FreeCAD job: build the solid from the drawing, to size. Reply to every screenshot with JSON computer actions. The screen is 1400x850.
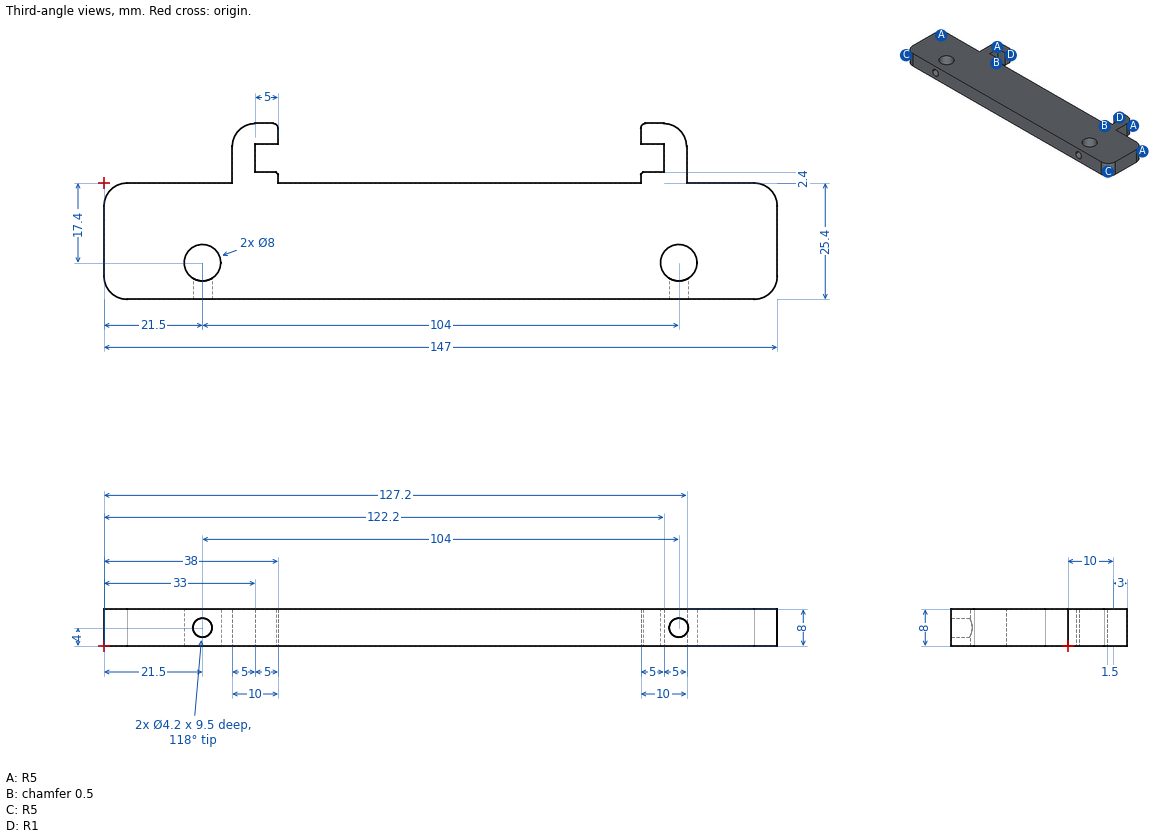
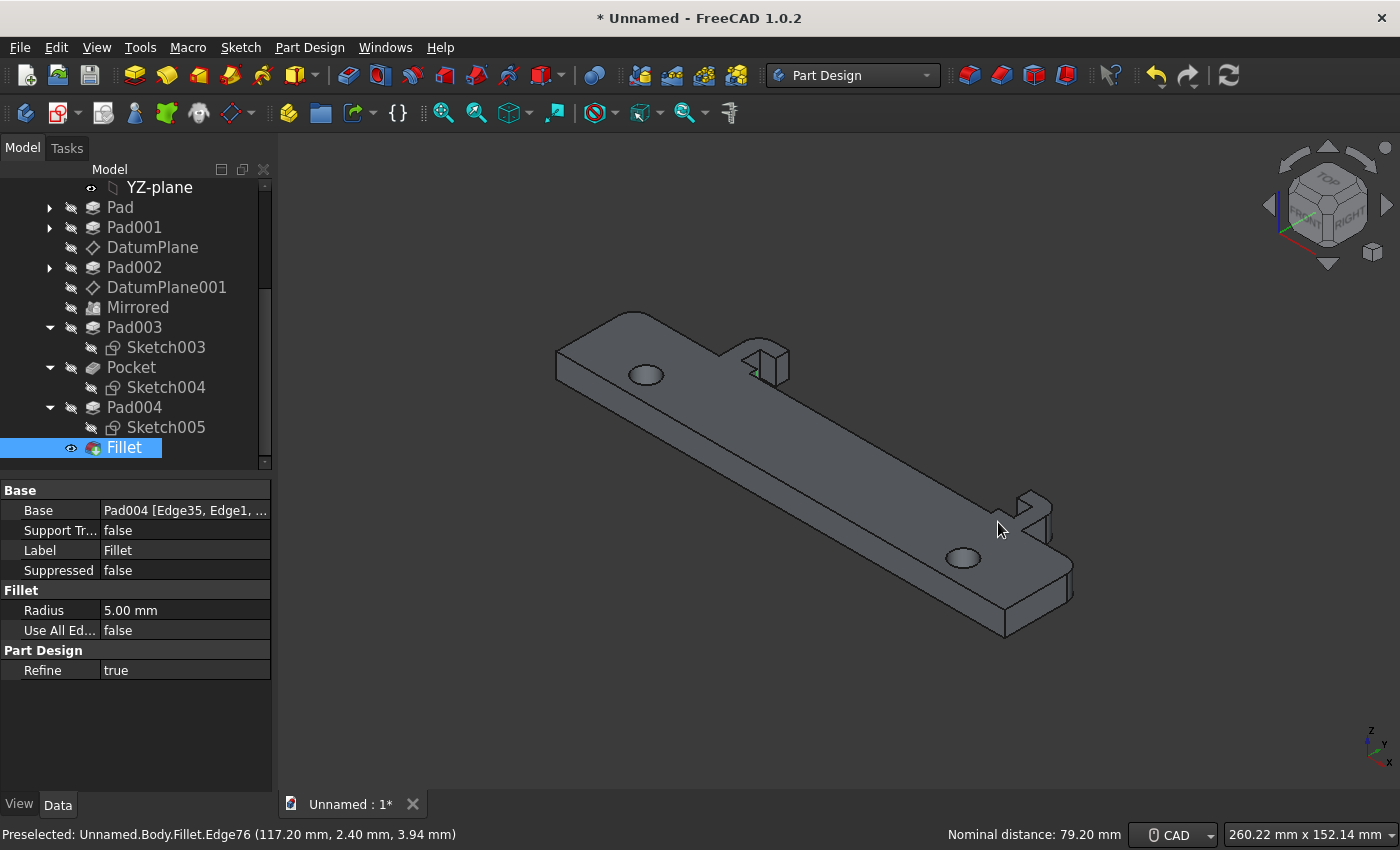
{"action": "left_click", "coordinate": [1002, 76]}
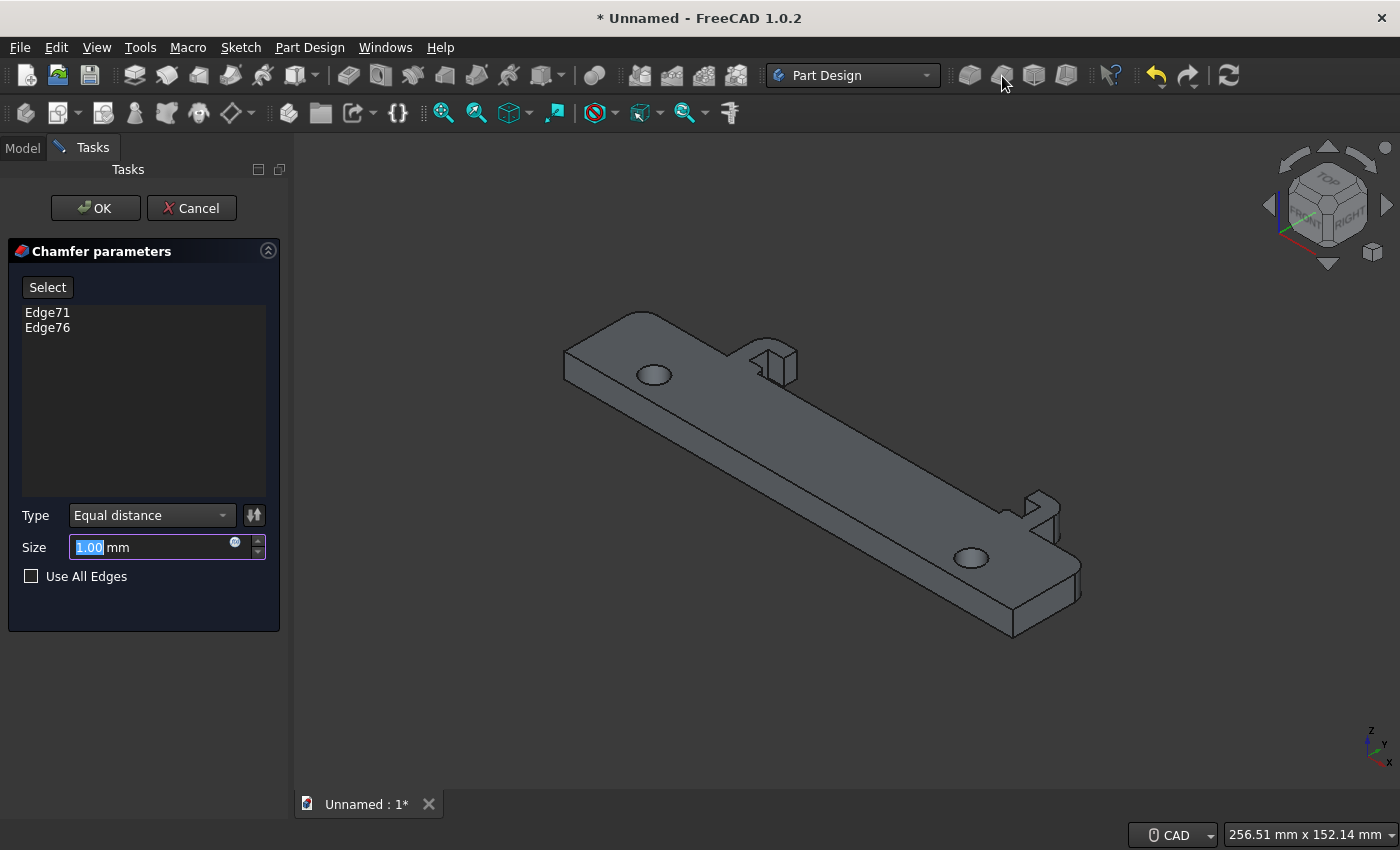
{"action": "type", "text": "0.5"}
{"action": "key", "text": "Tab"}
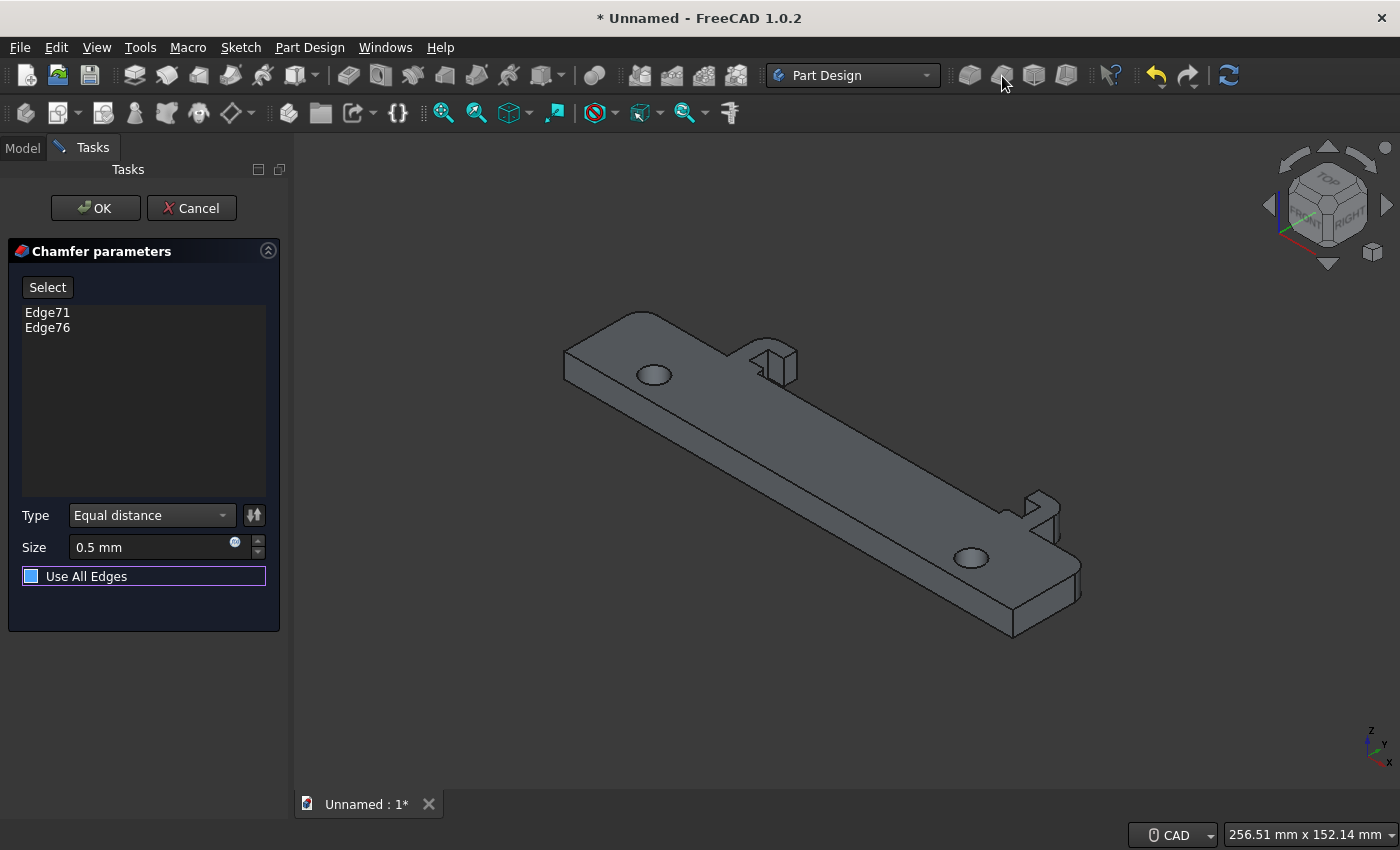
{"action": "left_click", "coordinate": [96, 208]}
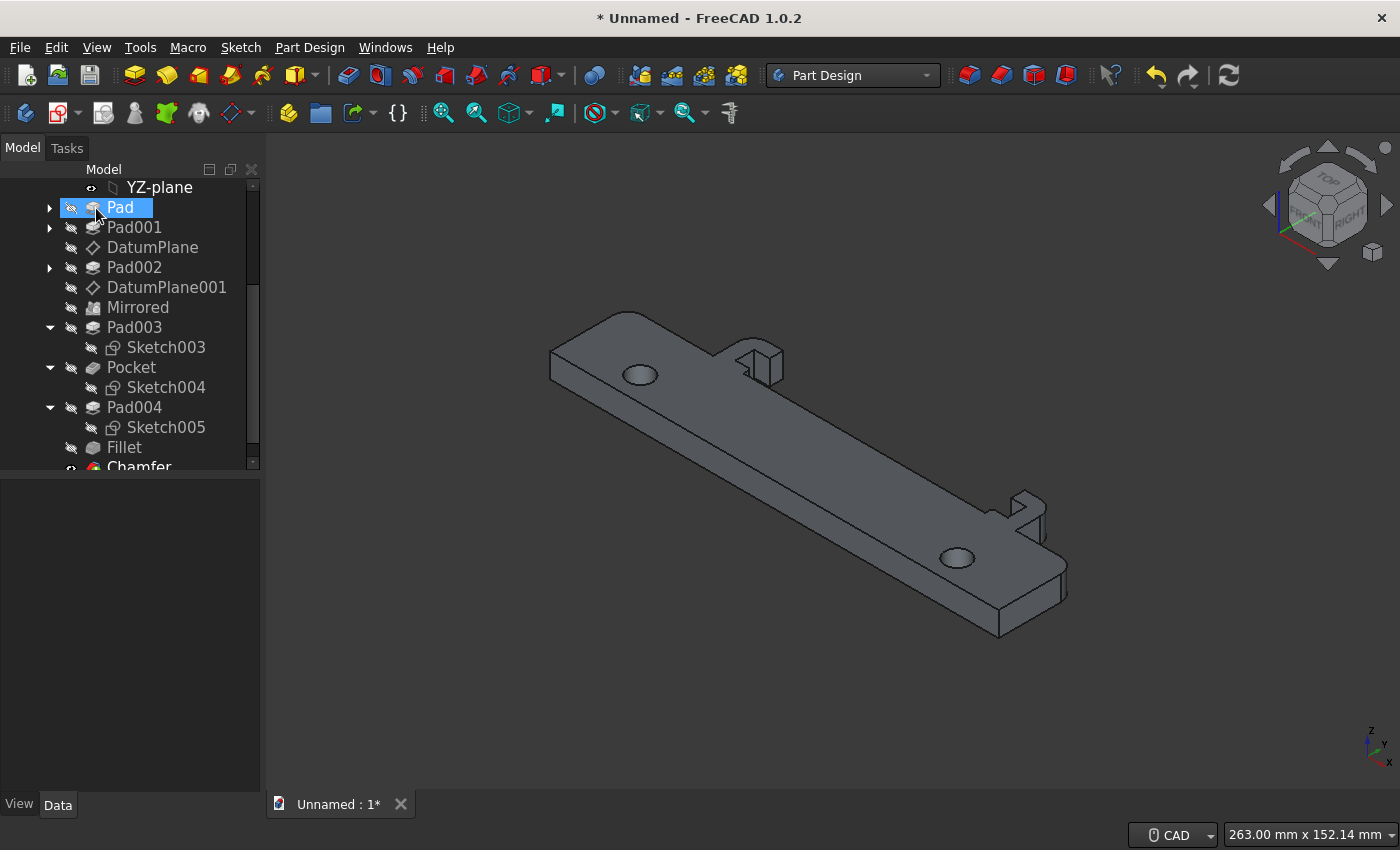
{"action": "left_click", "coordinate": [967, 605]}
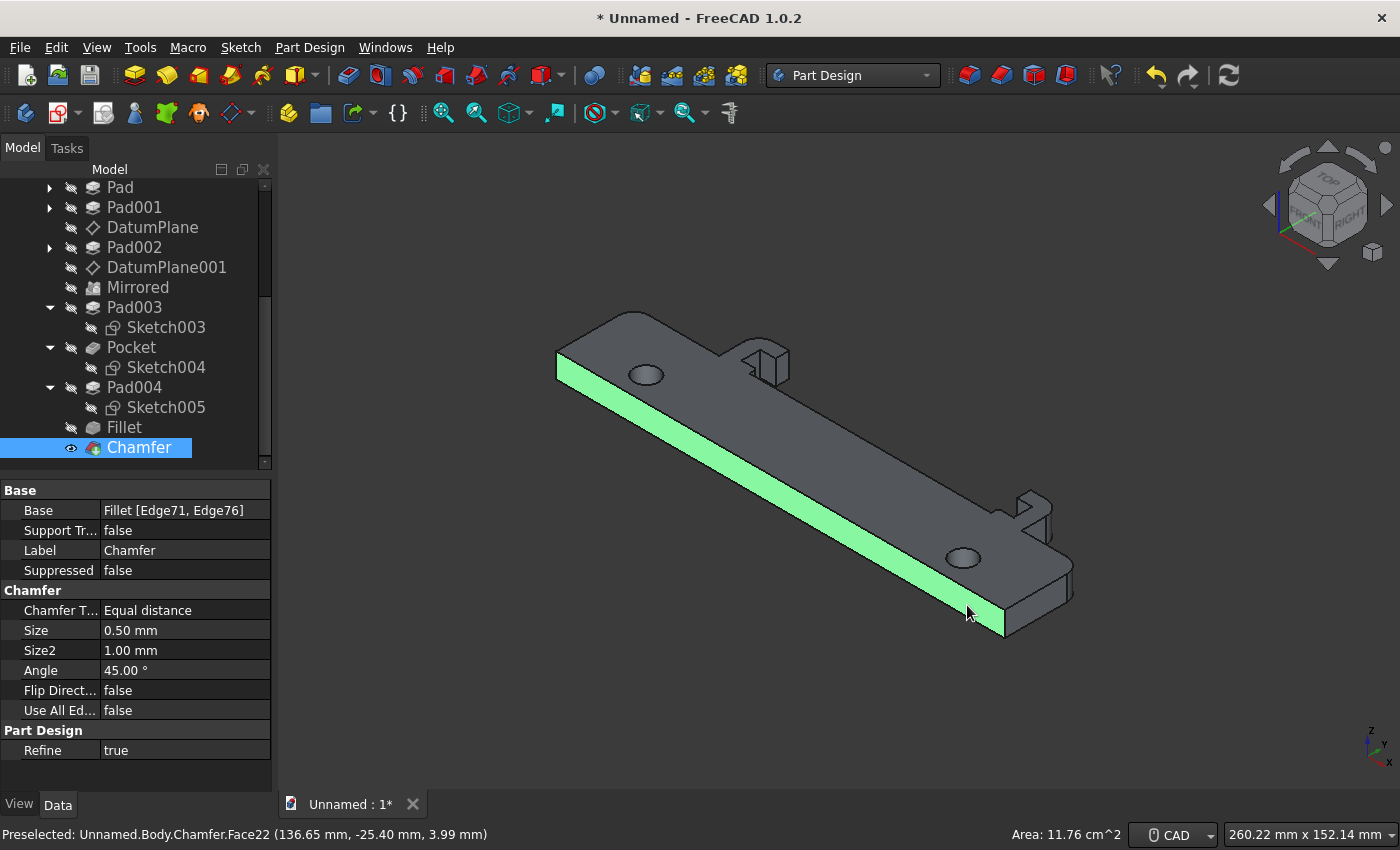
{"action": "left_click", "coordinate": [58, 114]}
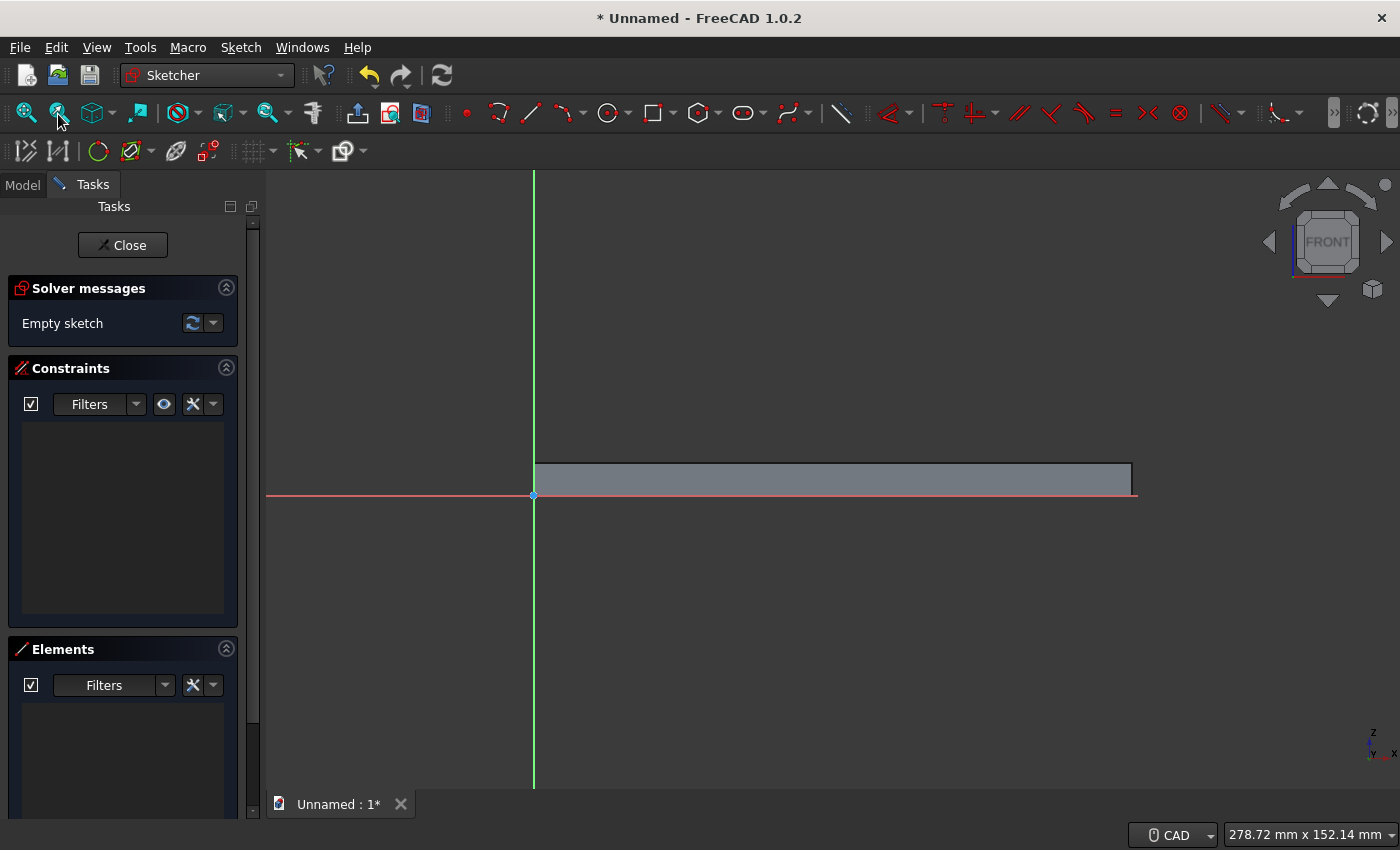
{"action": "left_click", "coordinate": [608, 114]}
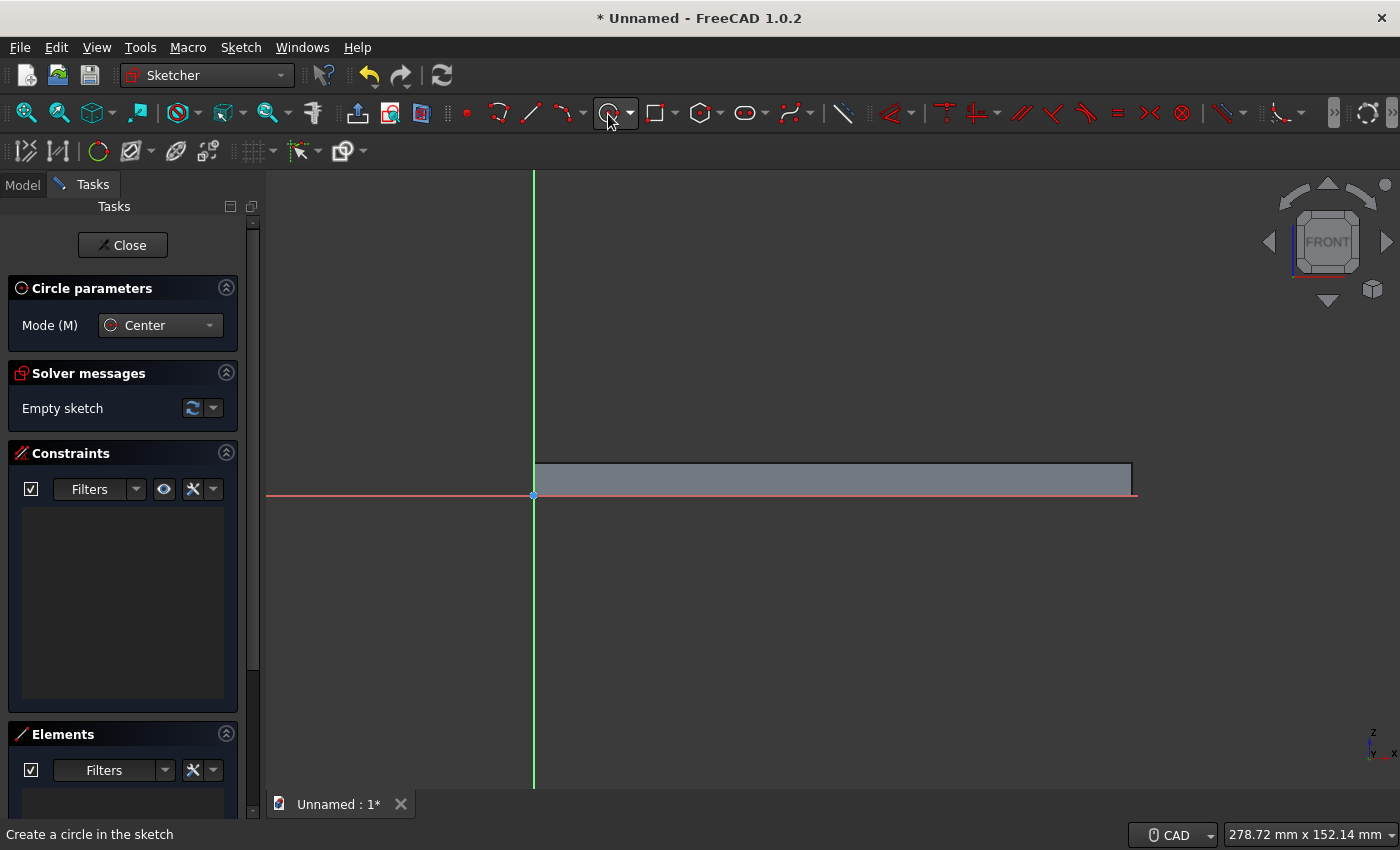
{"action": "scroll", "coordinate": [621, 480], "scroll_direction": "up", "scroll_amount": 5}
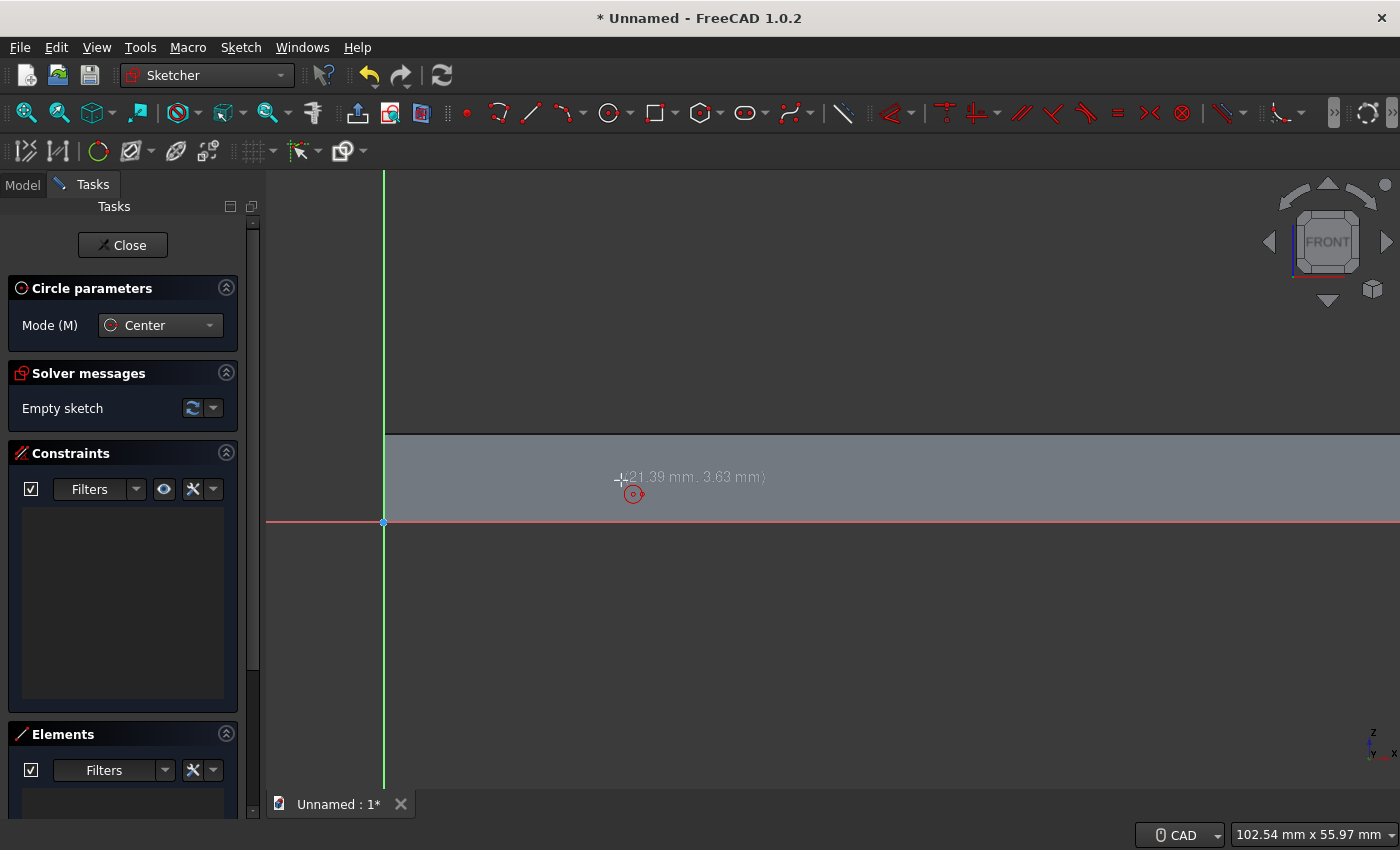
{"action": "left_click", "coordinate": [622, 478]}
{"action": "mouse_move", "coordinate": [638, 461]}